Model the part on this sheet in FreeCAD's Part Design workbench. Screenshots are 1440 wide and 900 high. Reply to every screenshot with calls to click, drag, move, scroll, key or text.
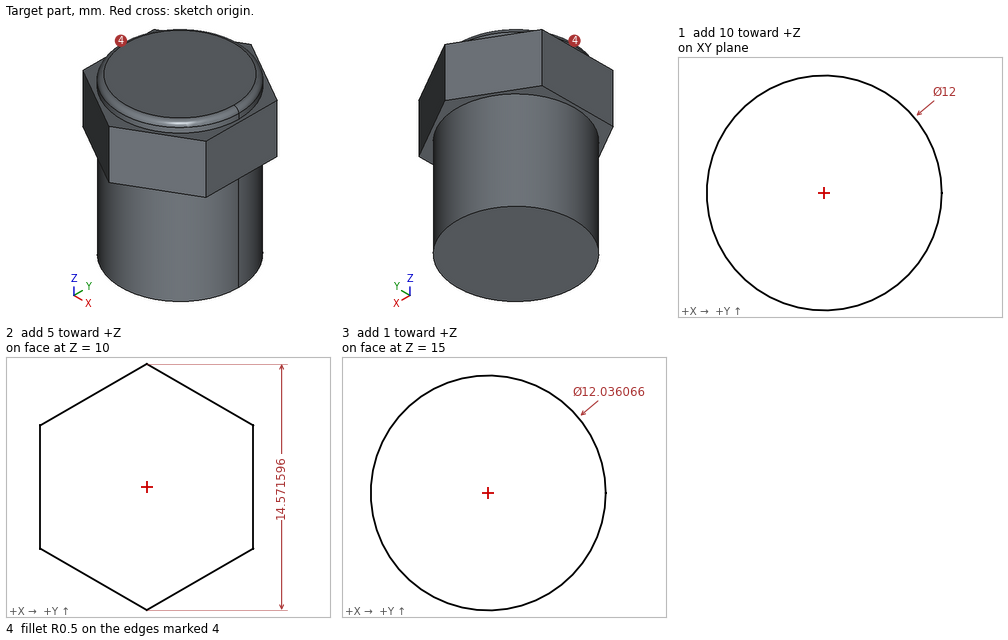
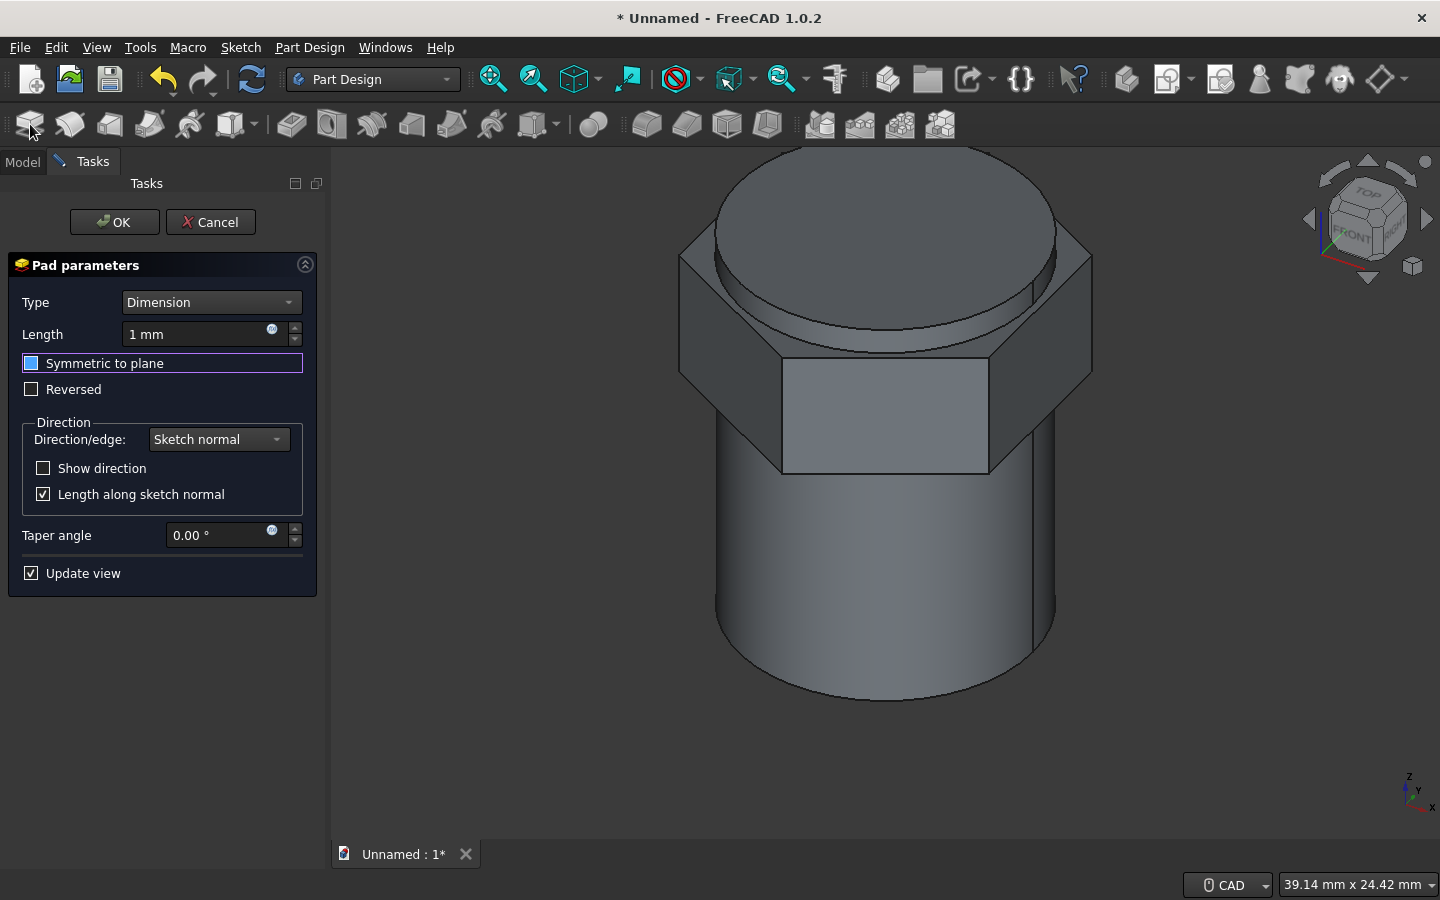
click(115, 222)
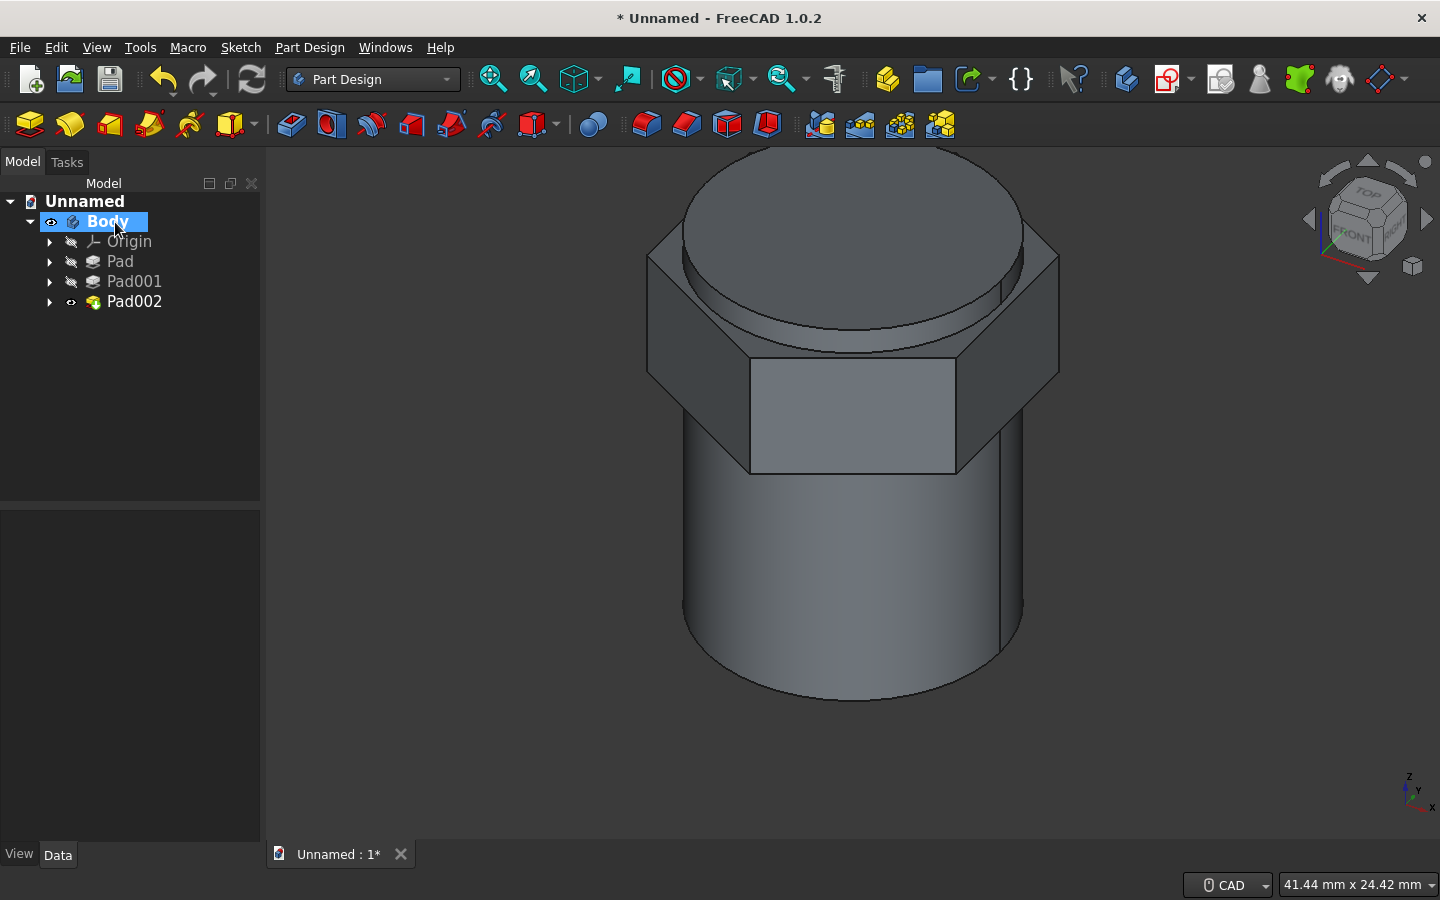
click(494, 80)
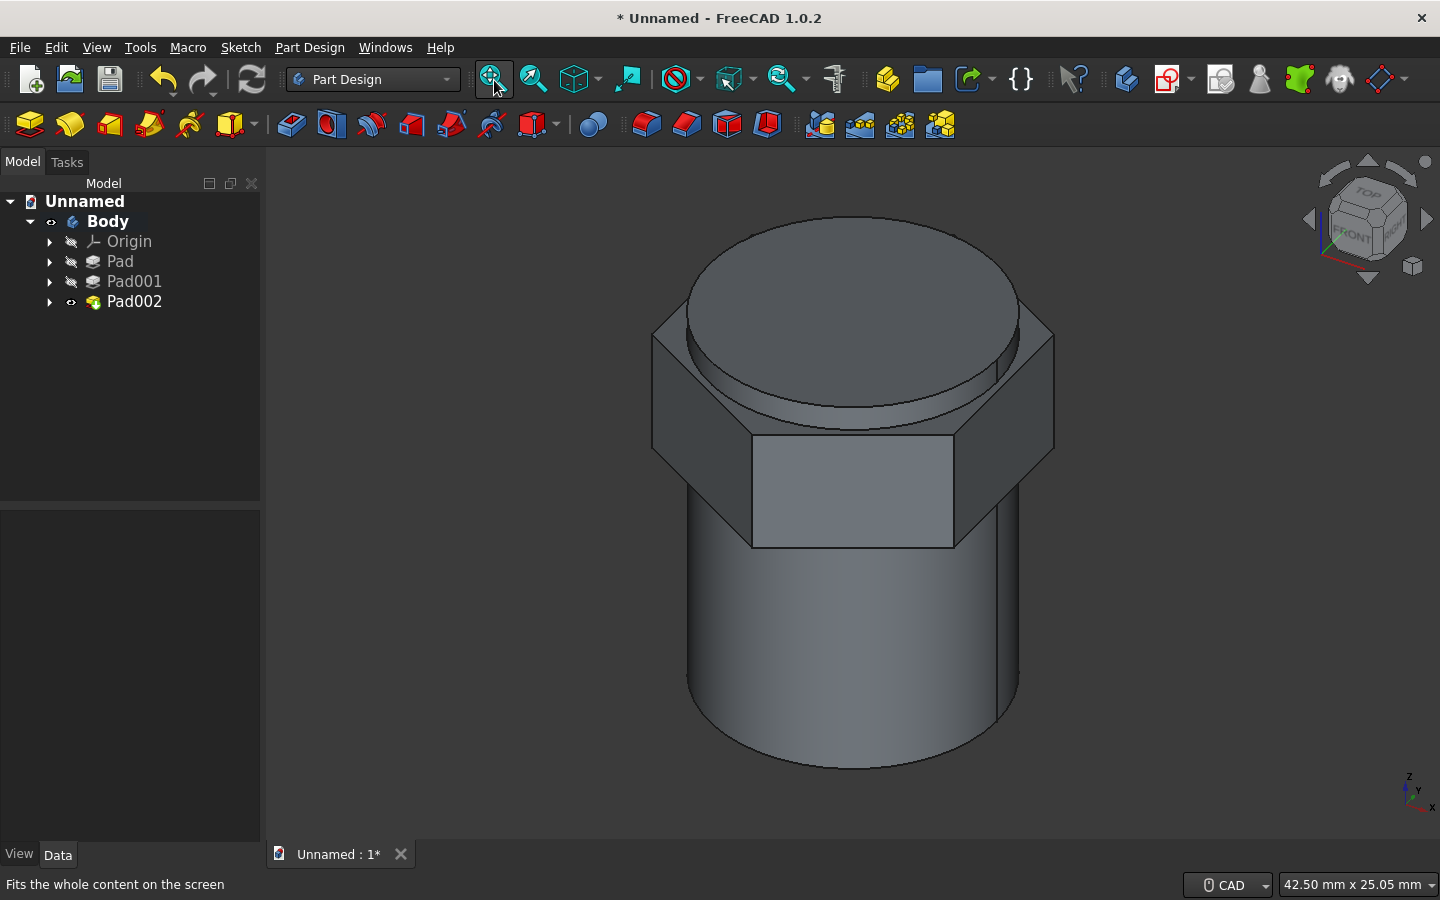
click(688, 321)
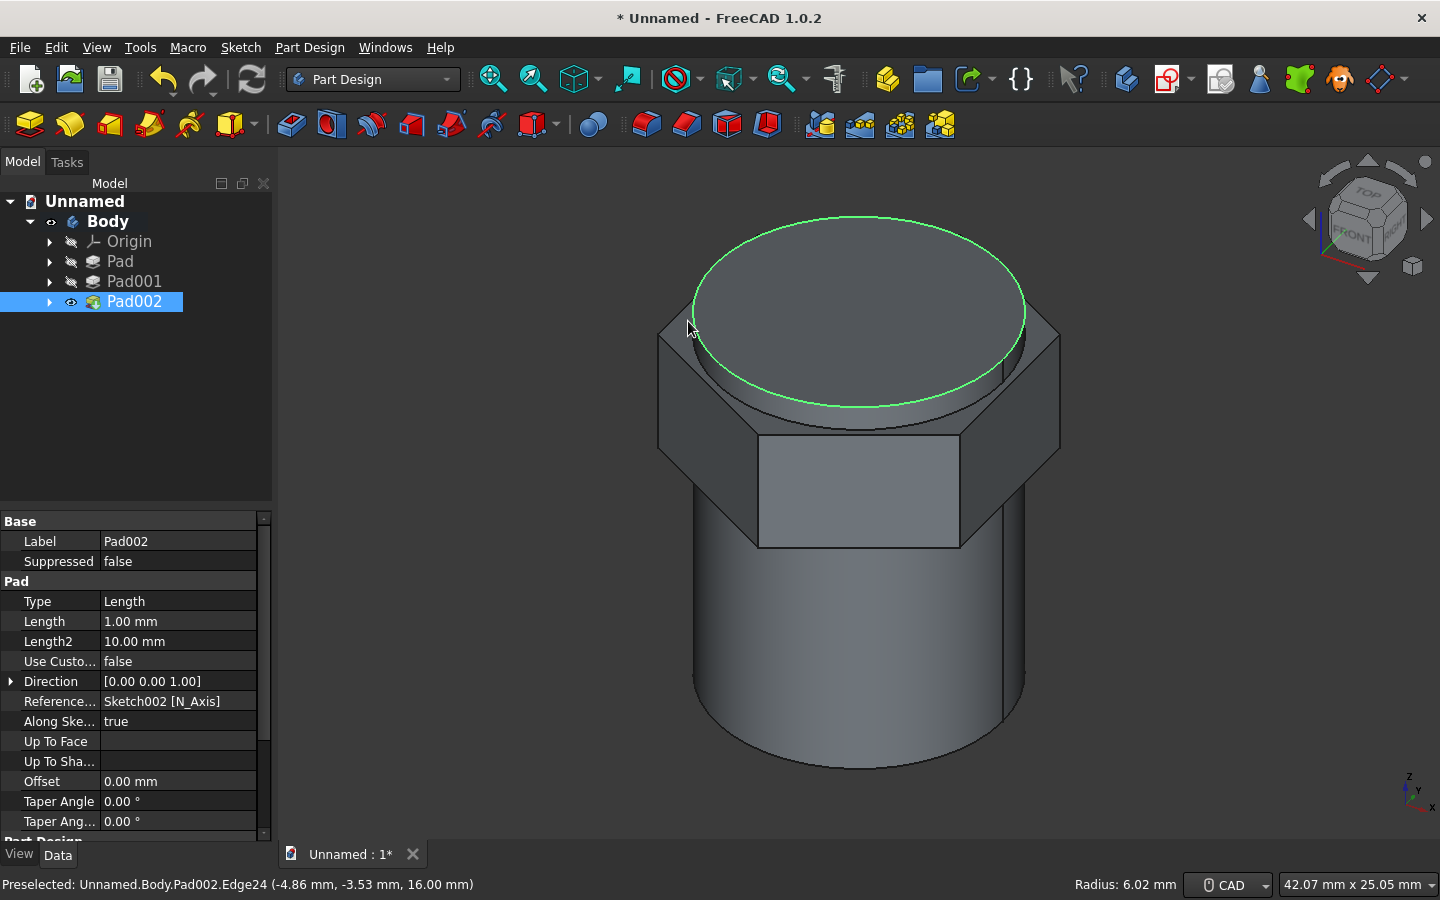
click(648, 124)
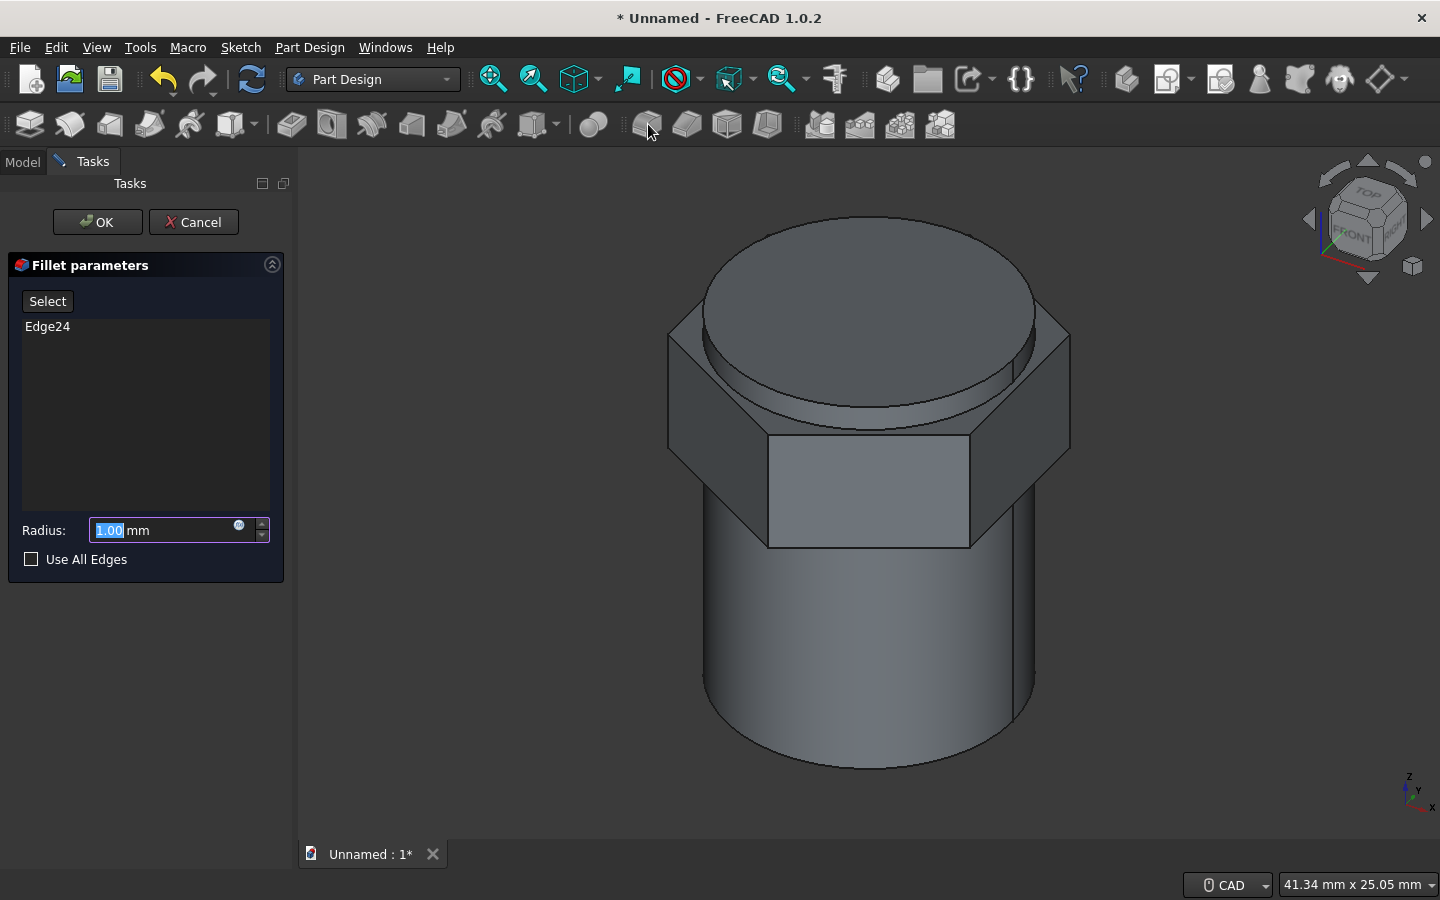
text(0.5)
key(Tab)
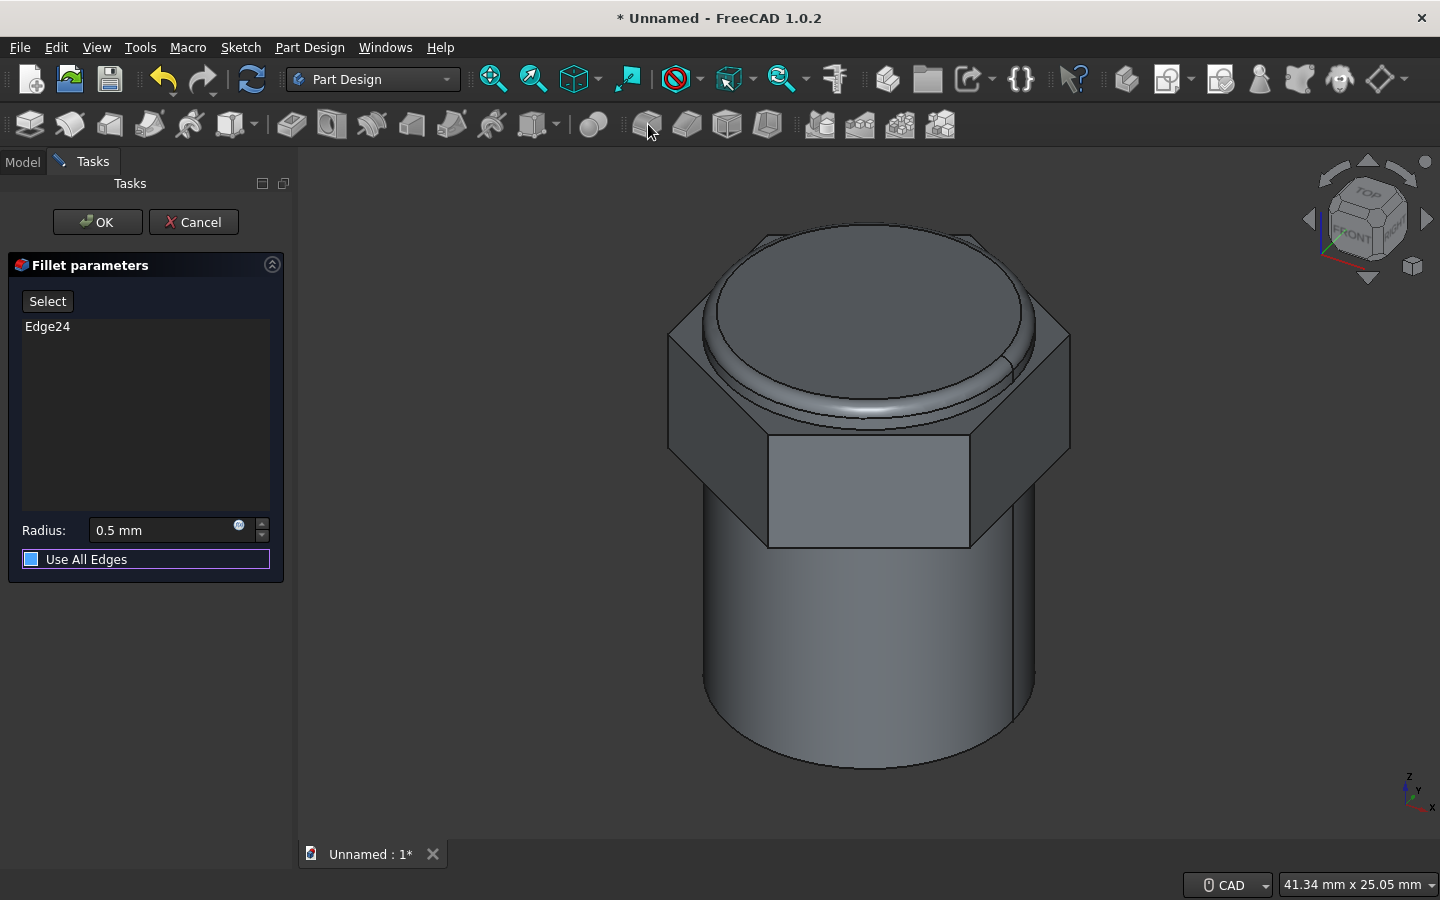
click(98, 222)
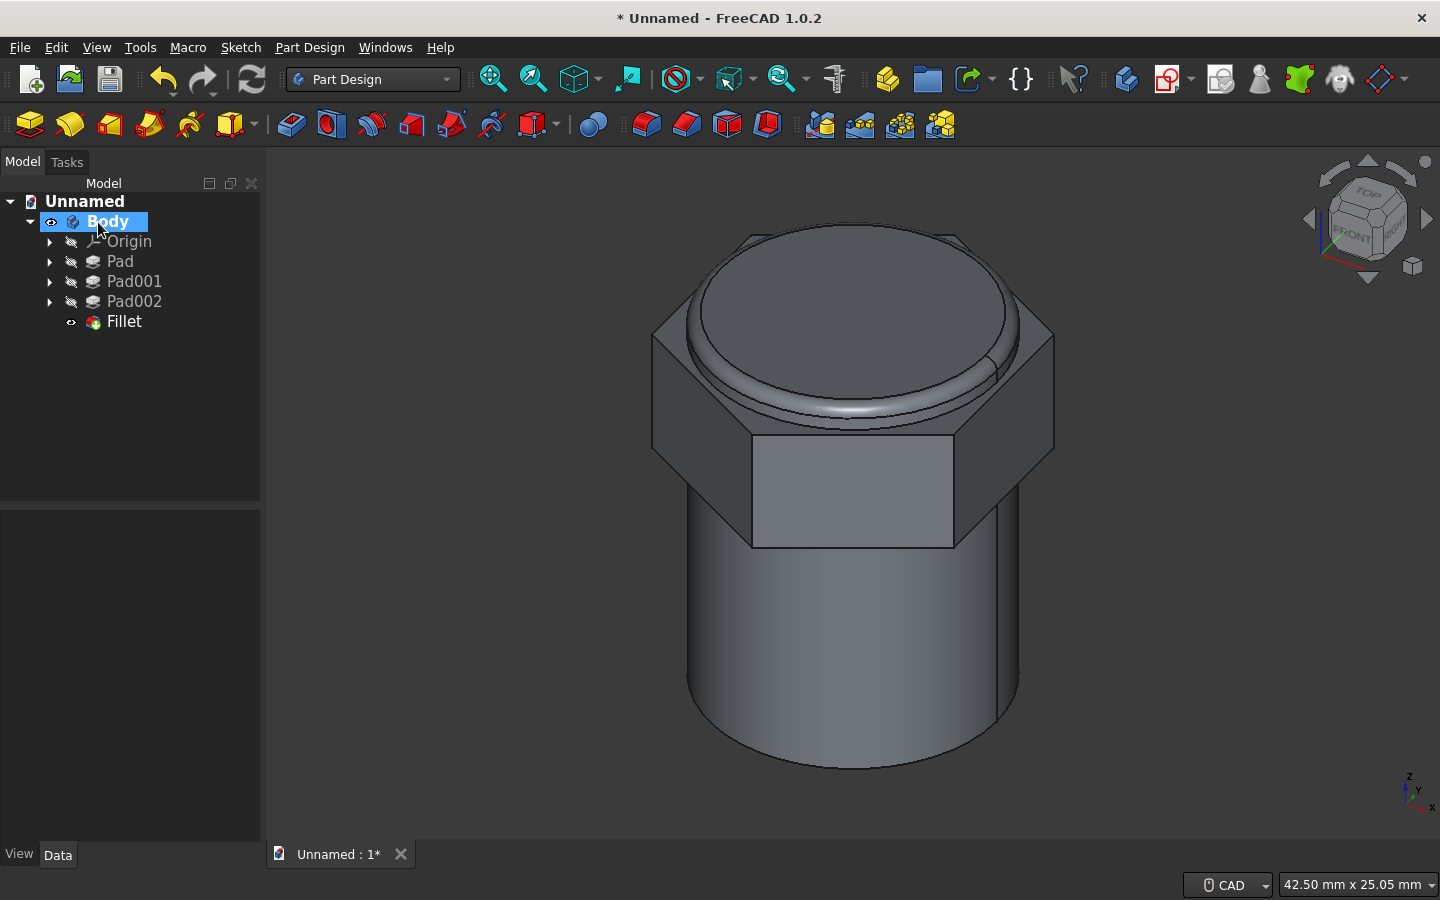
key(0)